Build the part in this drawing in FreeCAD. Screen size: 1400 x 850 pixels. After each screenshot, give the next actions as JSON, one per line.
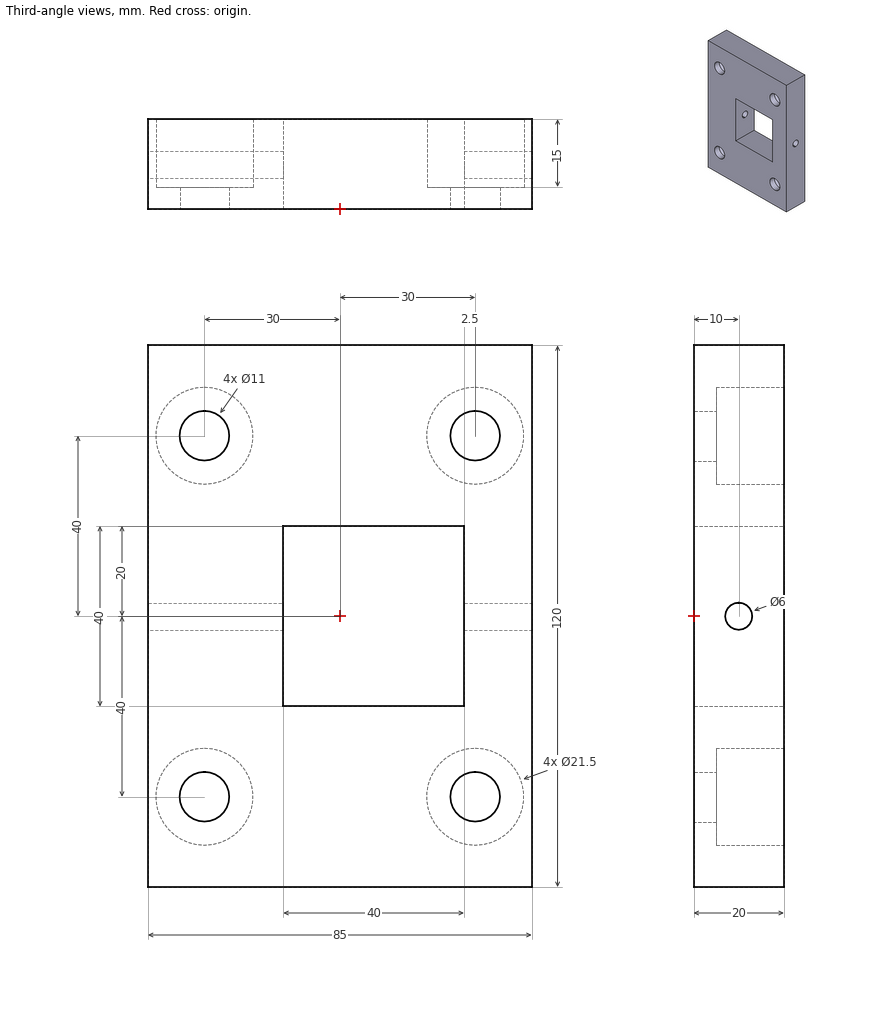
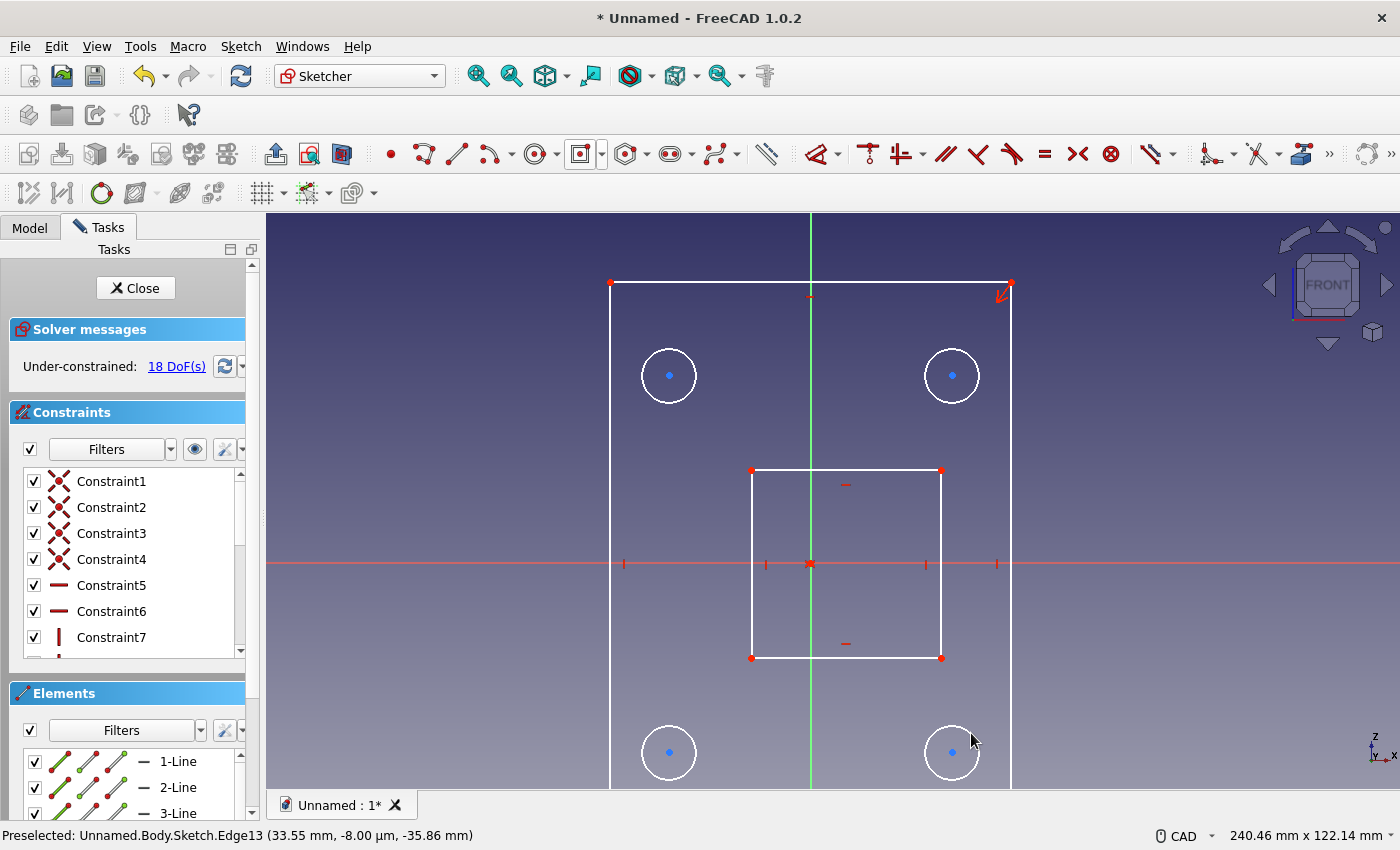
{"action": "left_click", "coordinate": [688, 357]}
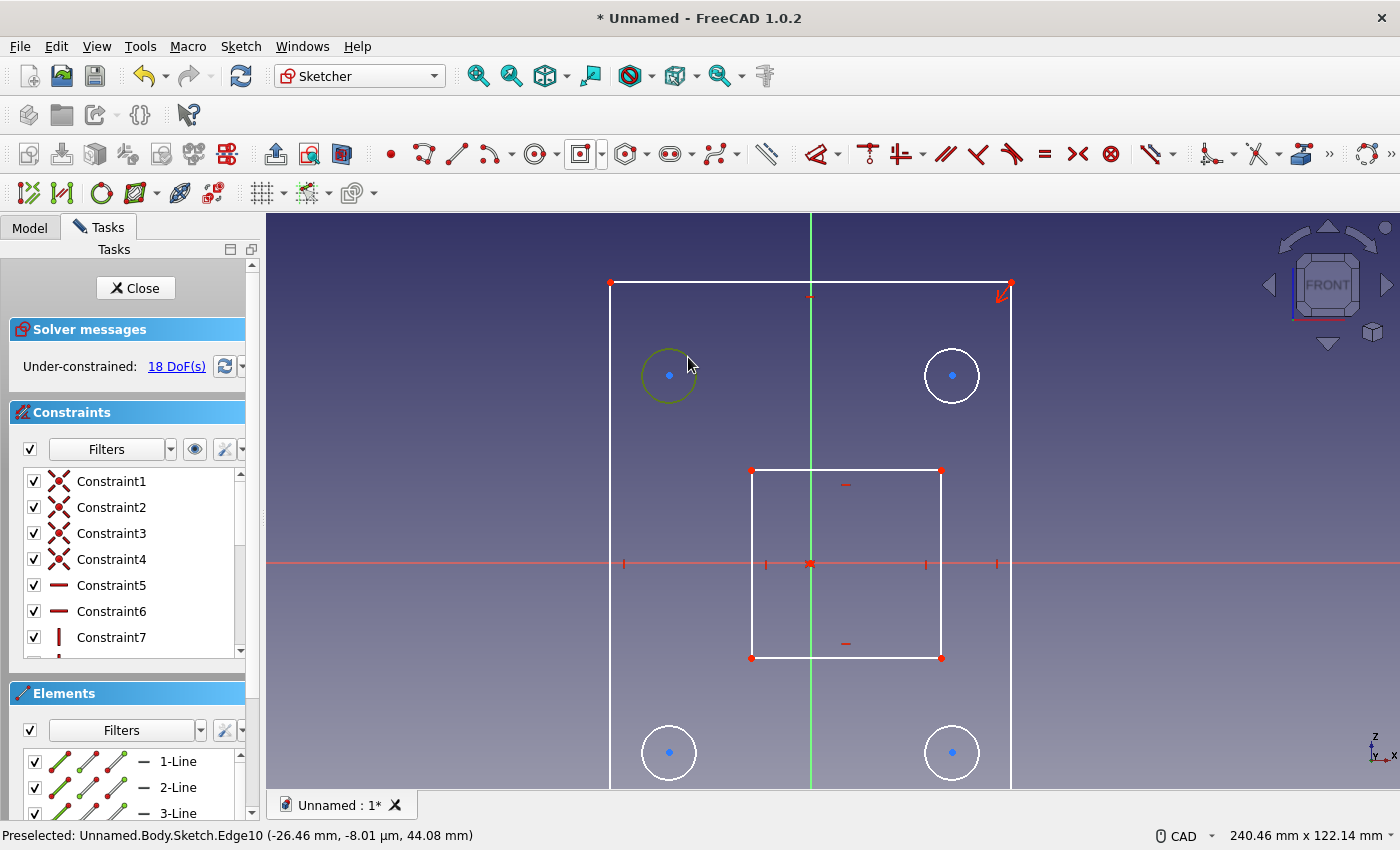
{"action": "left_click", "coordinate": [971, 357]}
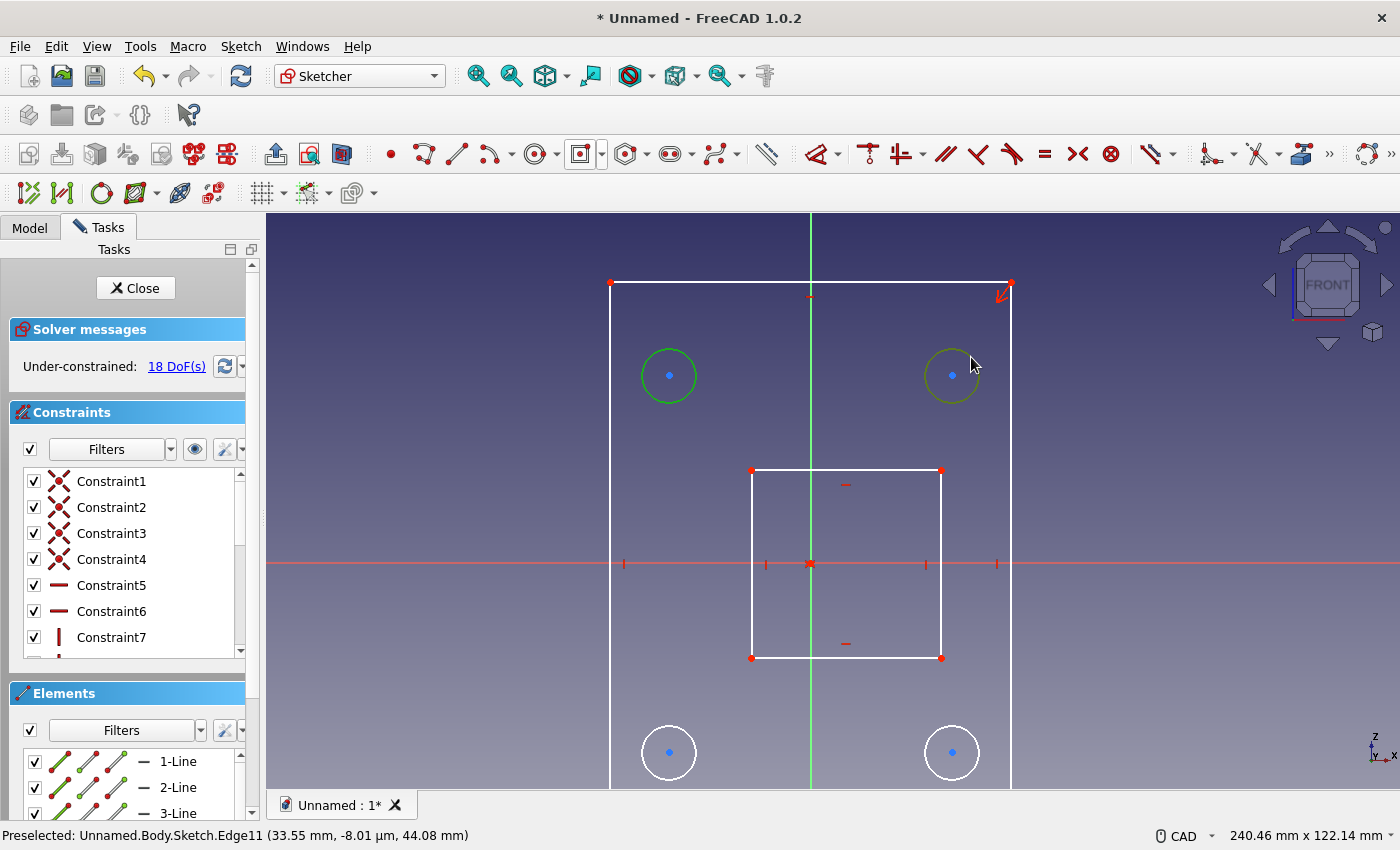
{"action": "left_click", "coordinate": [688, 734]}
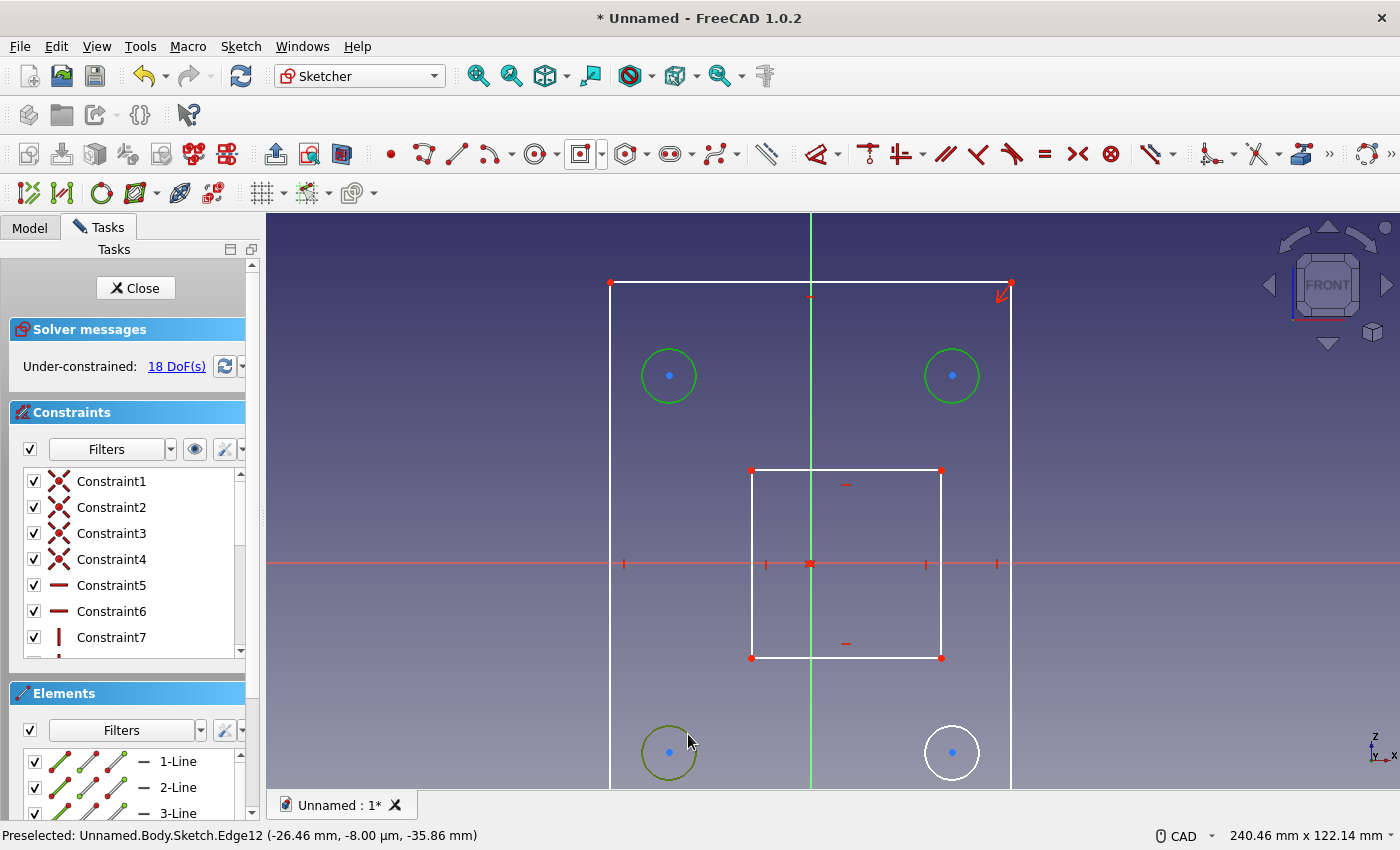
{"action": "left_click", "coordinate": [971, 734]}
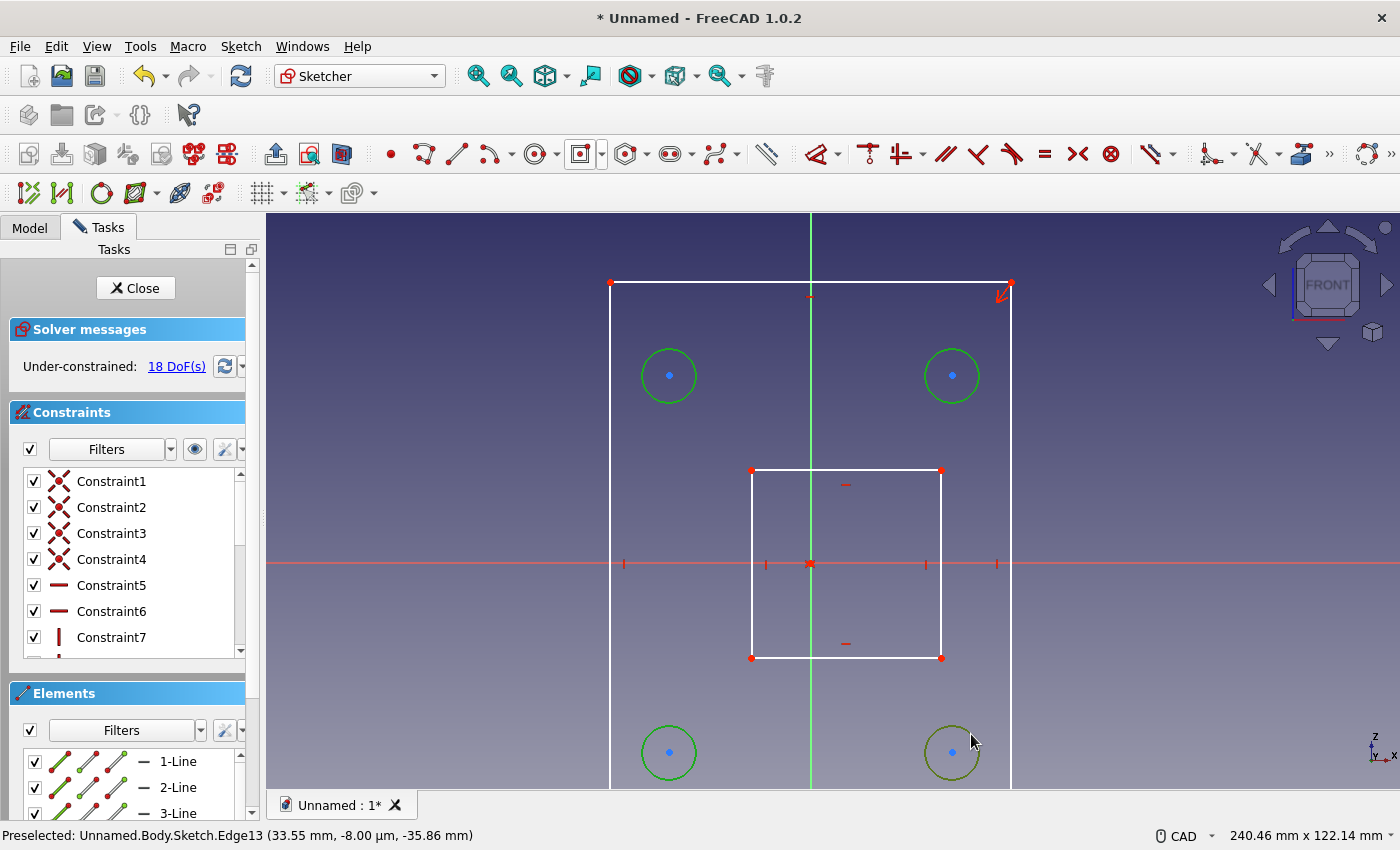
{"action": "key", "text": "e"}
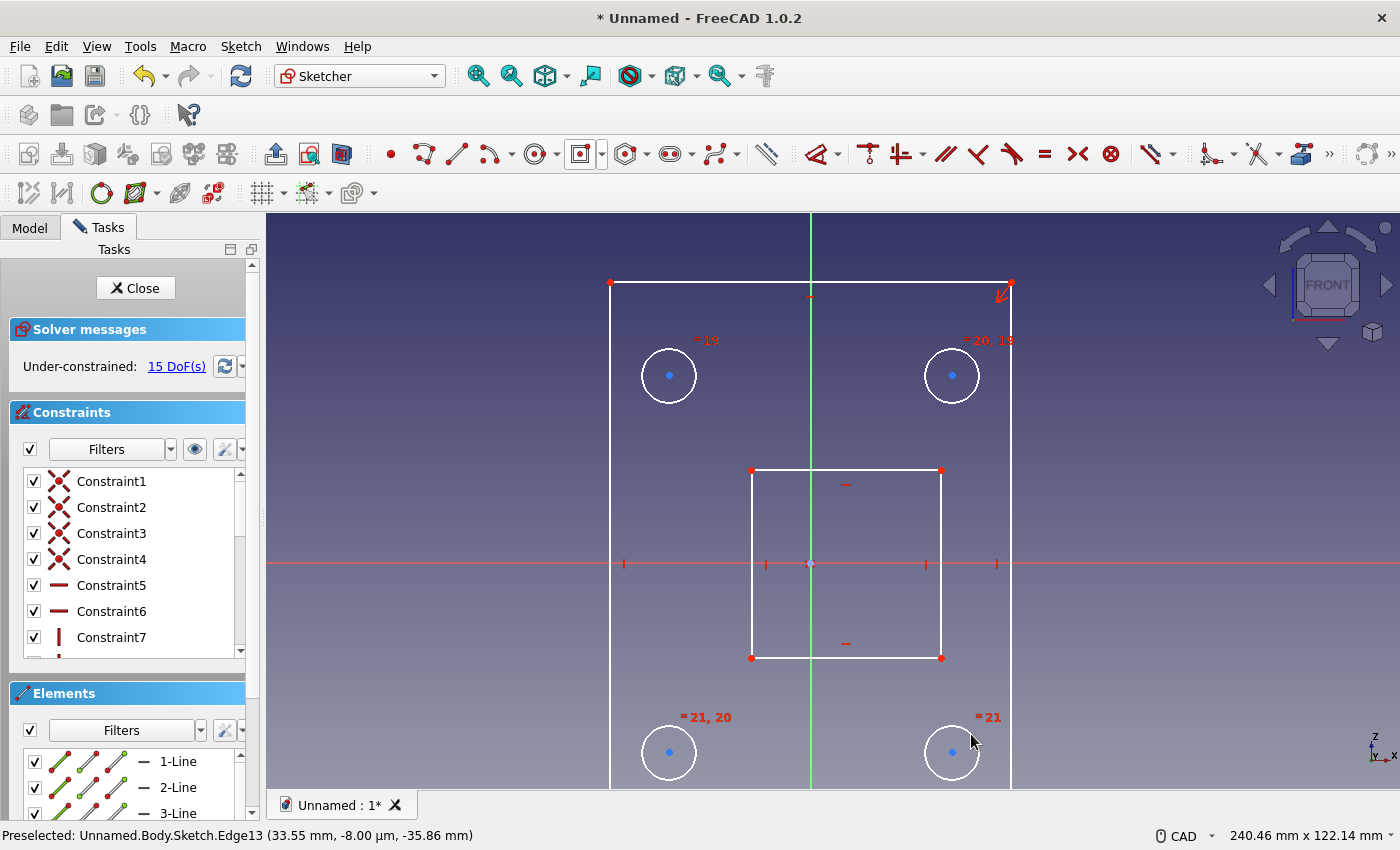
{"action": "key", "text": "d"}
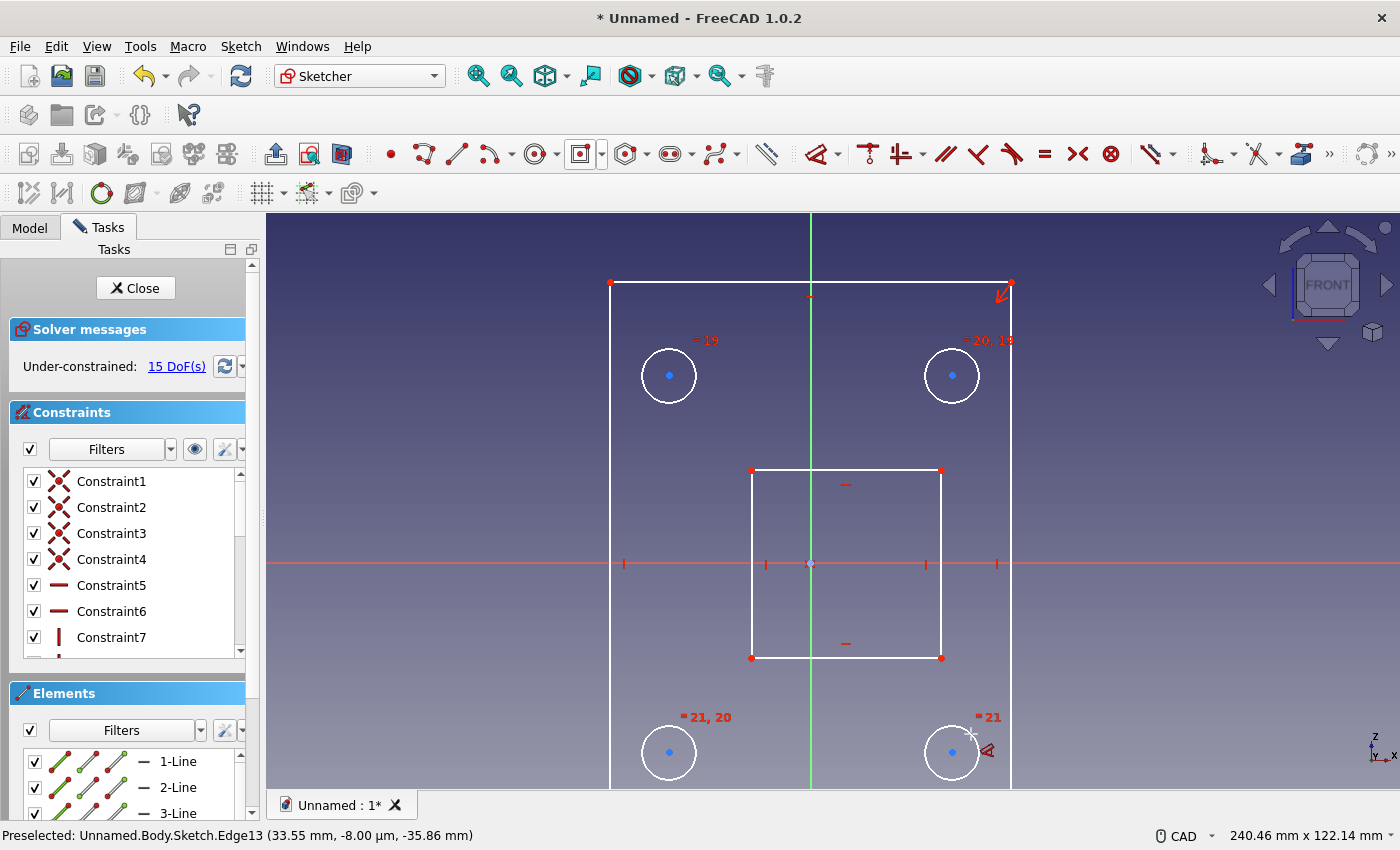
{"action": "left_click", "coordinate": [688, 357]}
{"action": "left_click", "coordinate": [711, 334]}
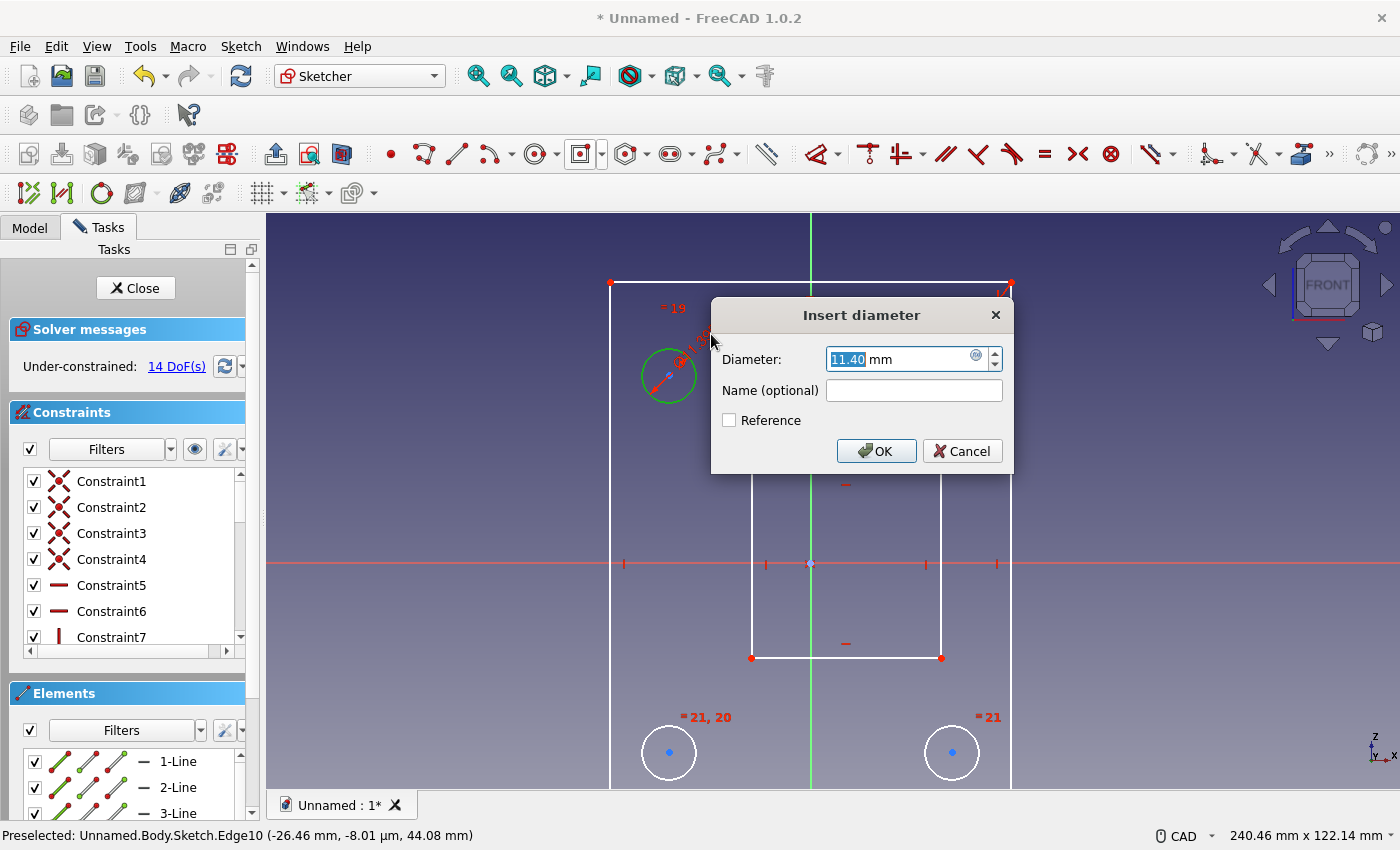
{"action": "type", "text": "11"}
{"action": "key", "text": "Return"}